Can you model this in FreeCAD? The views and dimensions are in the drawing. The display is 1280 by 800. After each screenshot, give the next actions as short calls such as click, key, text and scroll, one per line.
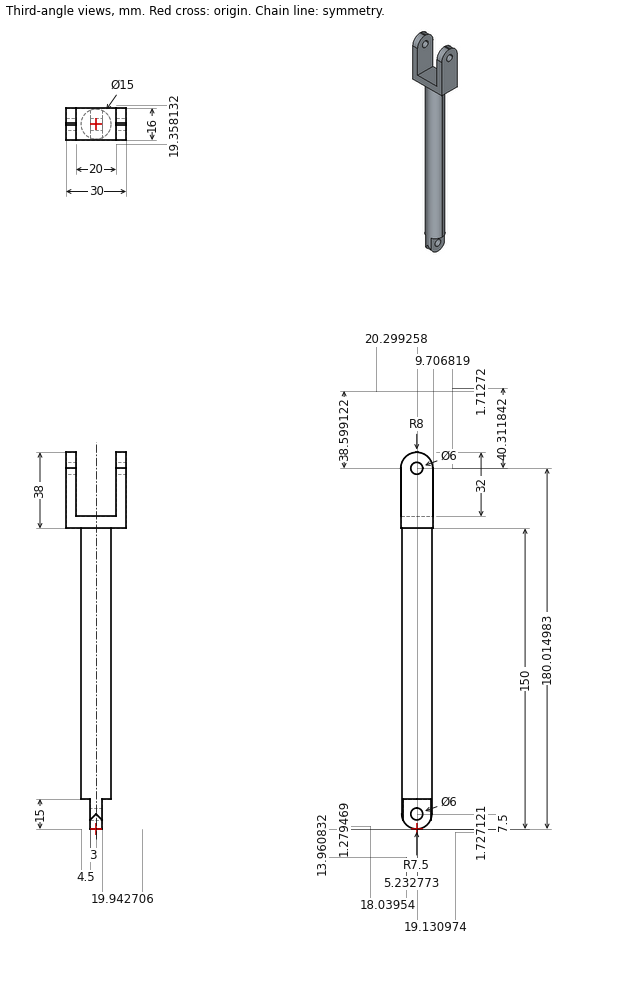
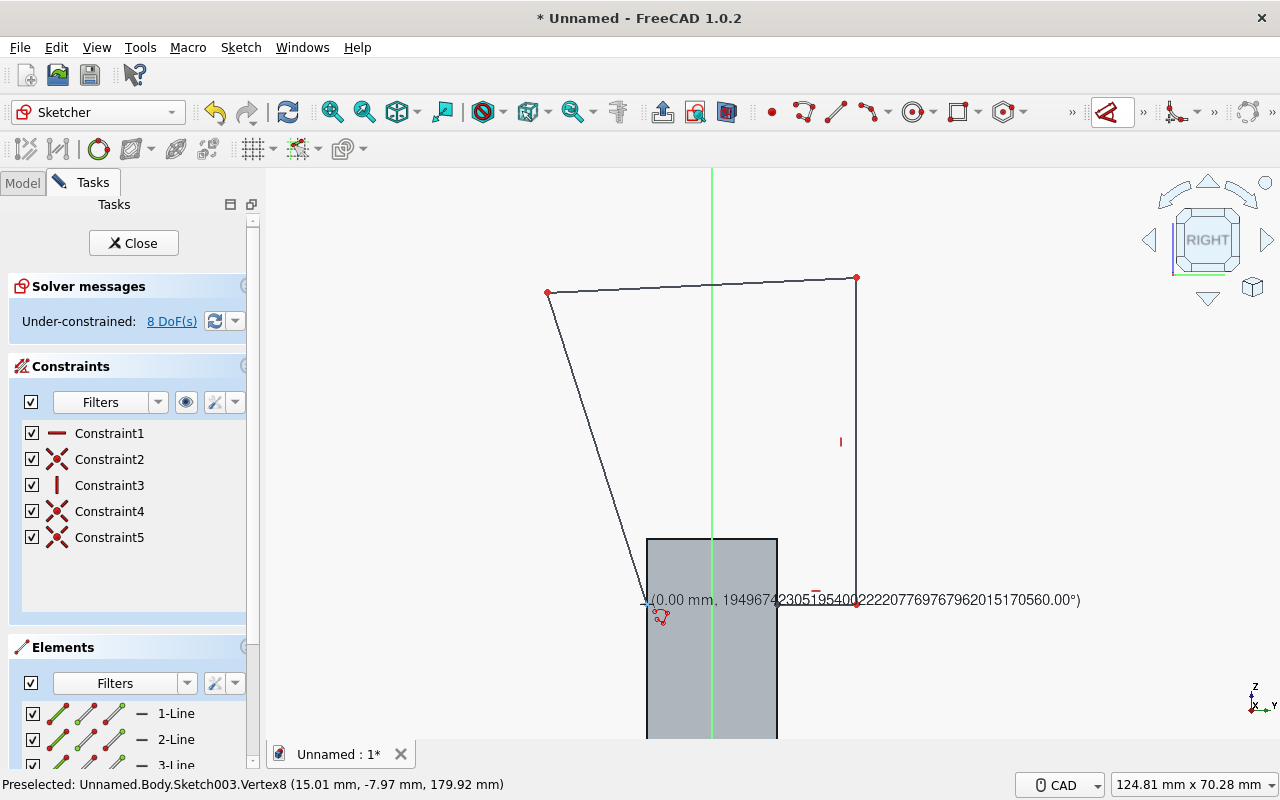
click(868, 112)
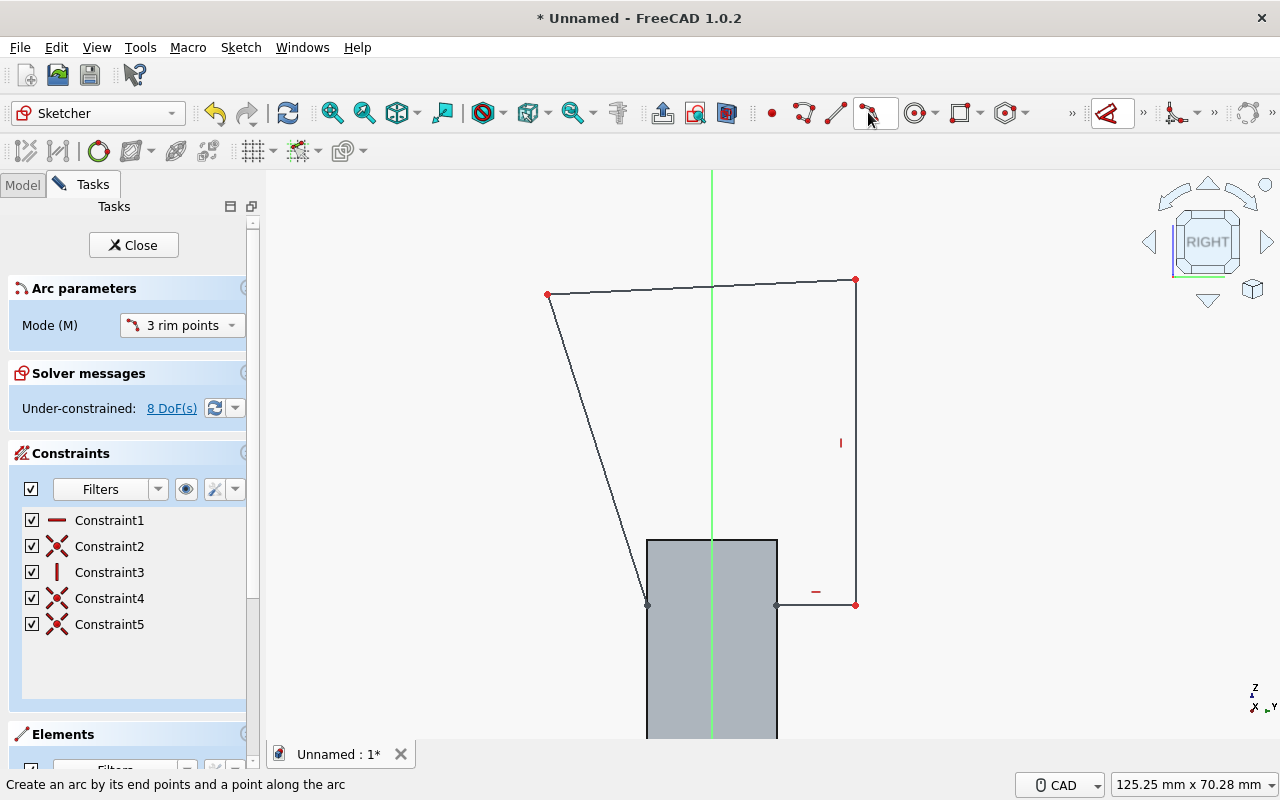
click(647, 605)
click(777, 605)
click(732, 543)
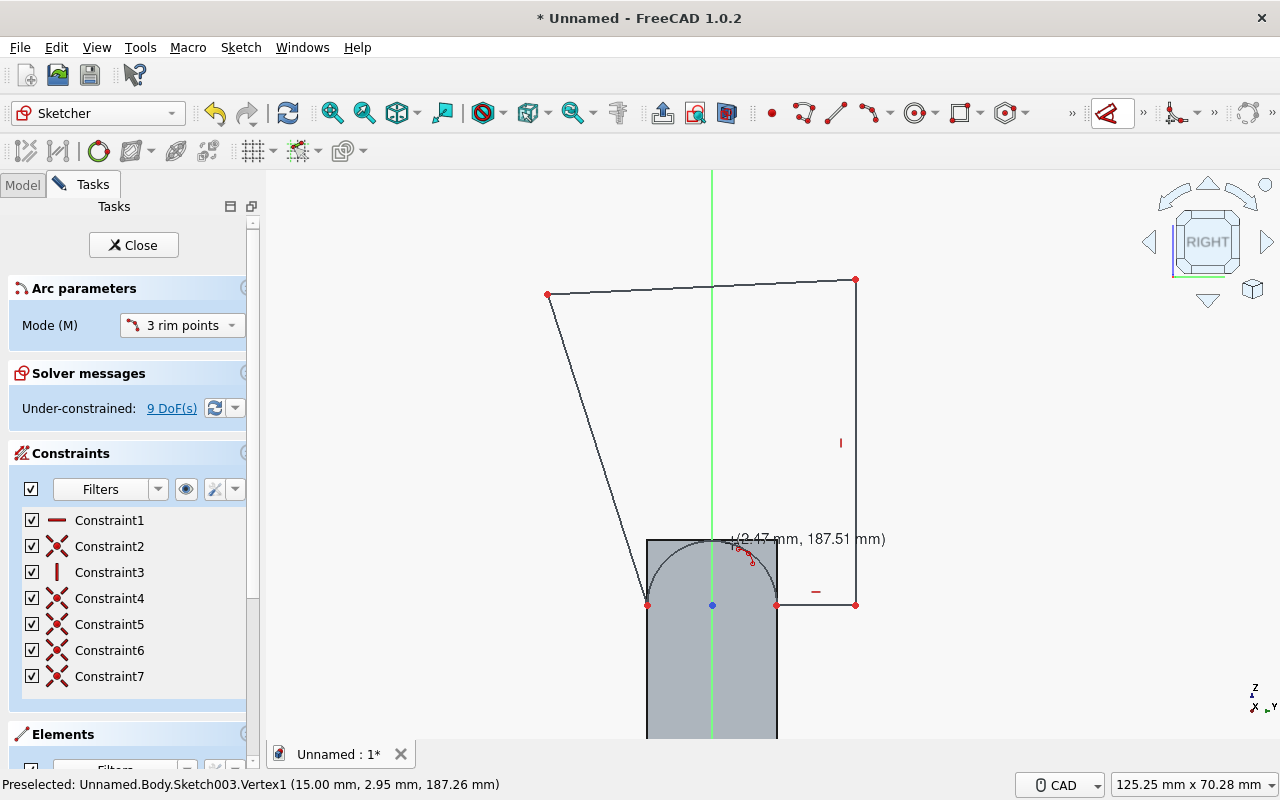
click(916, 114)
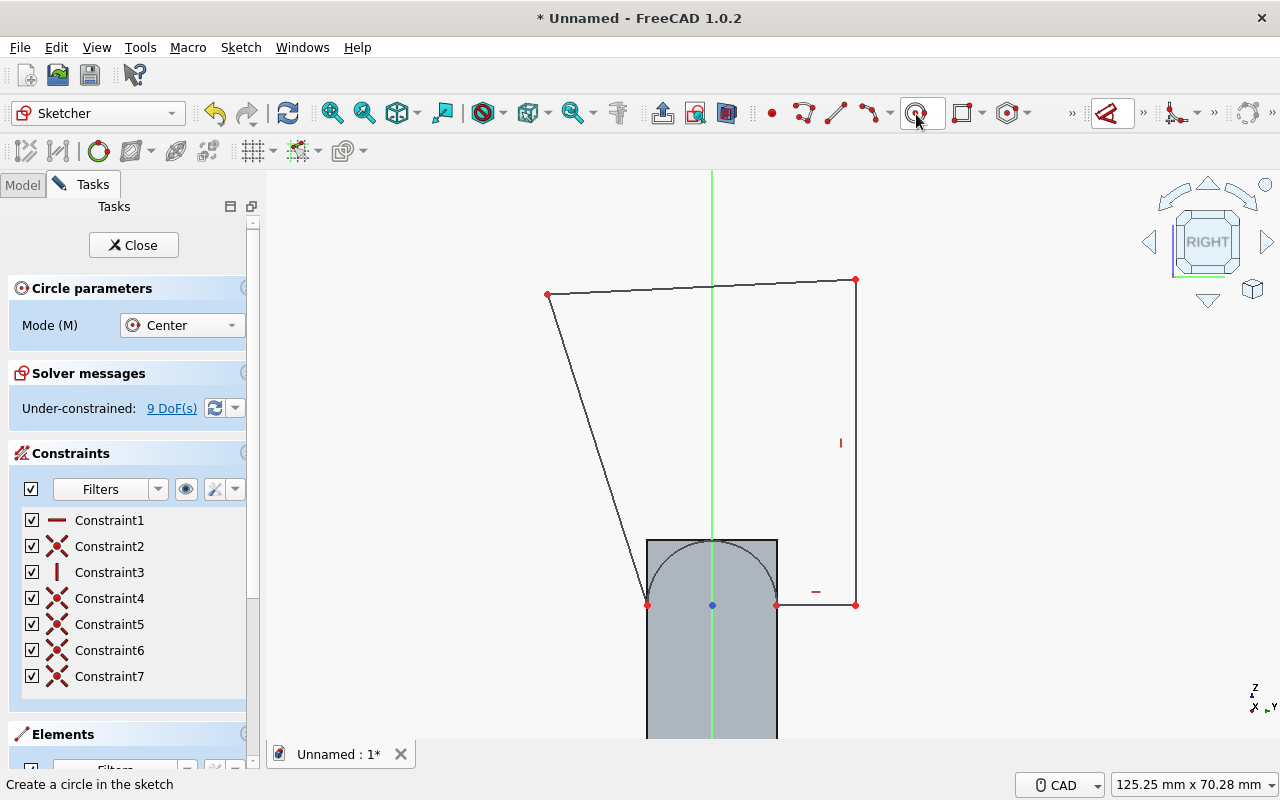
click(712, 605)
move(729, 588)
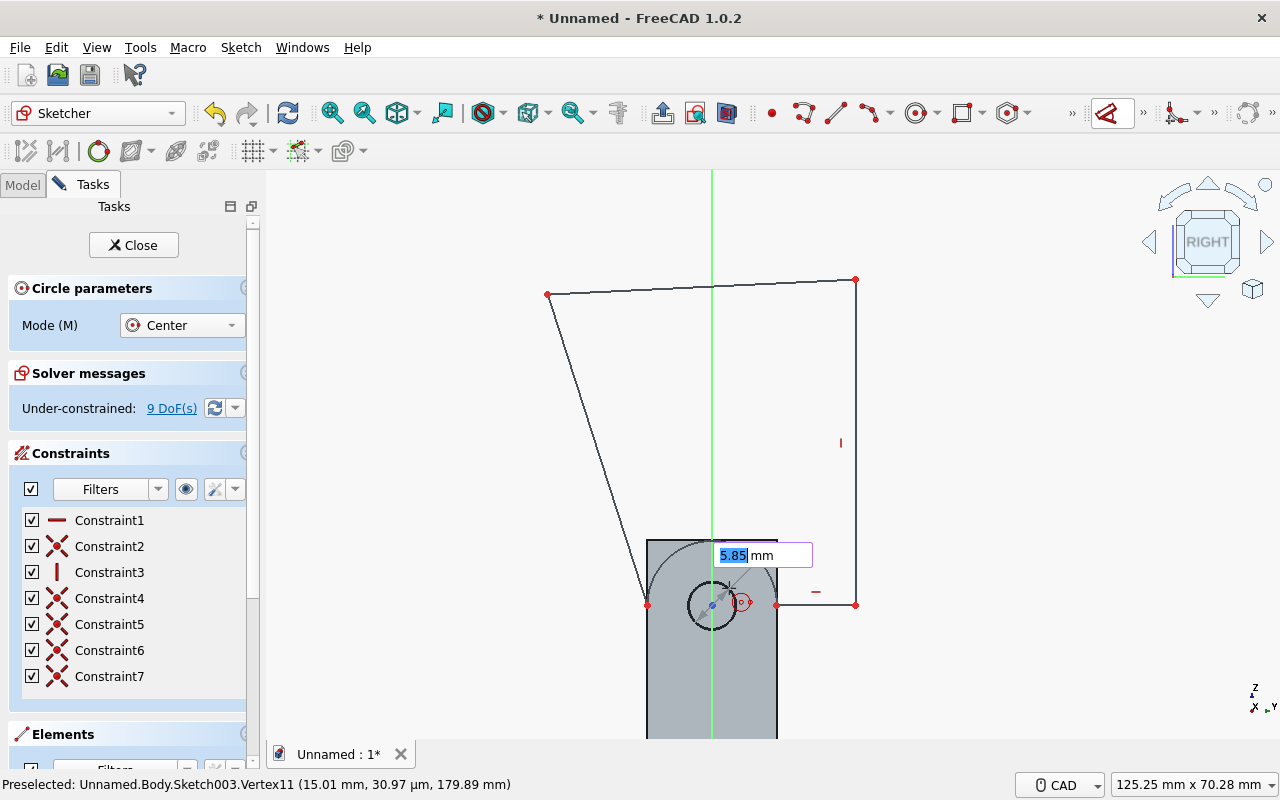
text(6)
key(Return)
key(Escape)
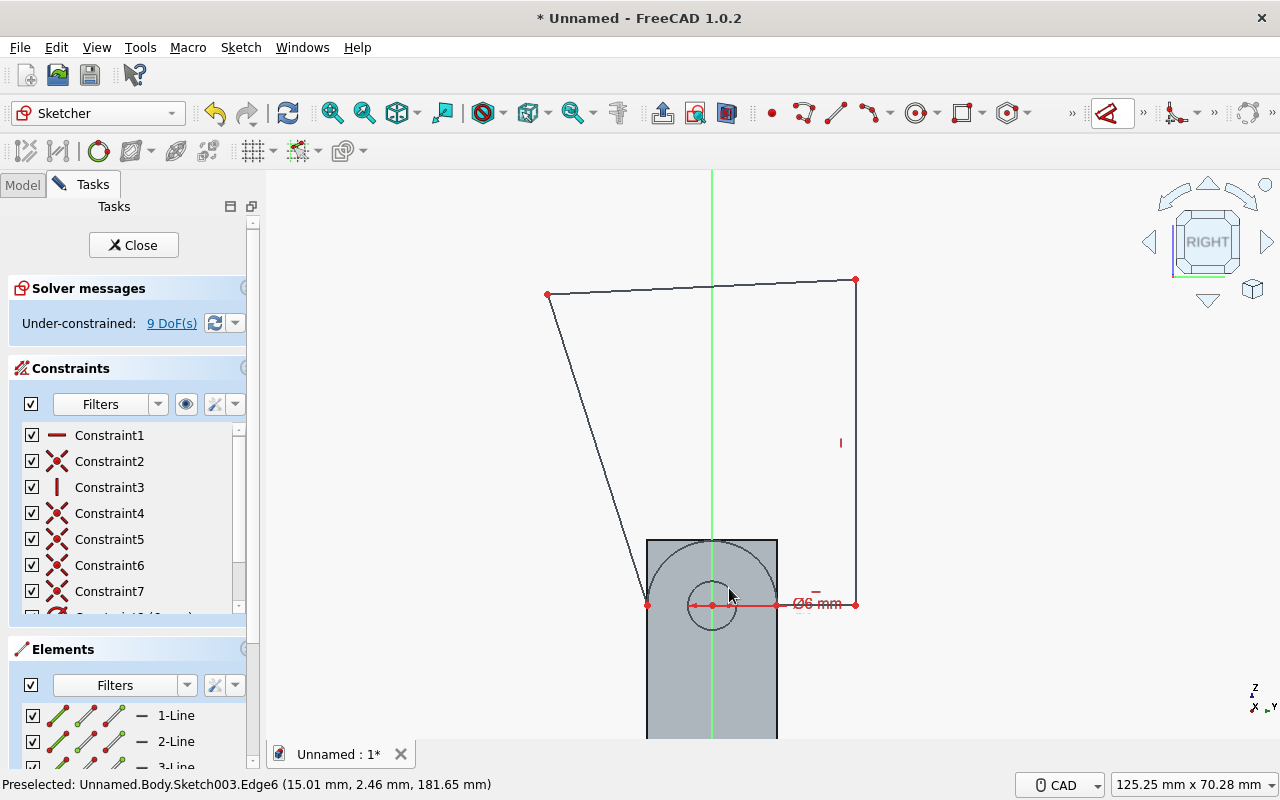
click(712, 606)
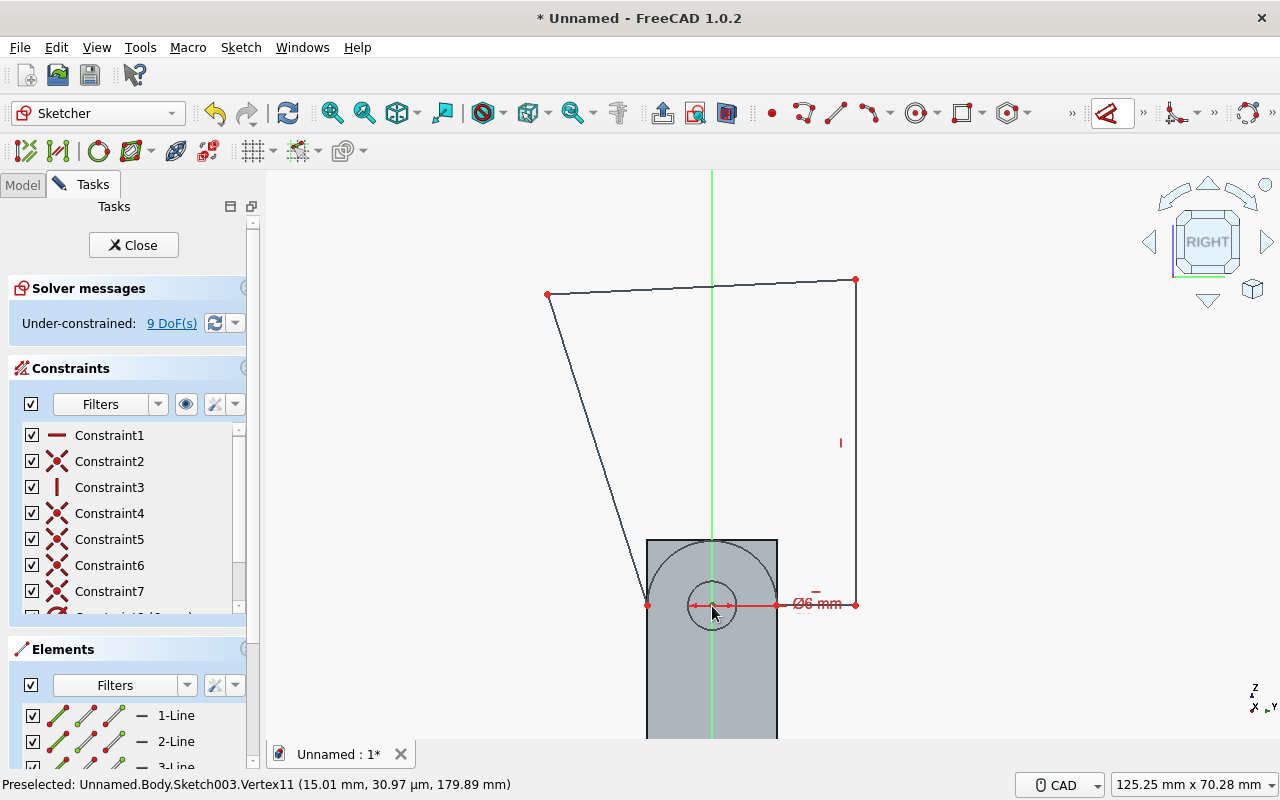
click(712, 674)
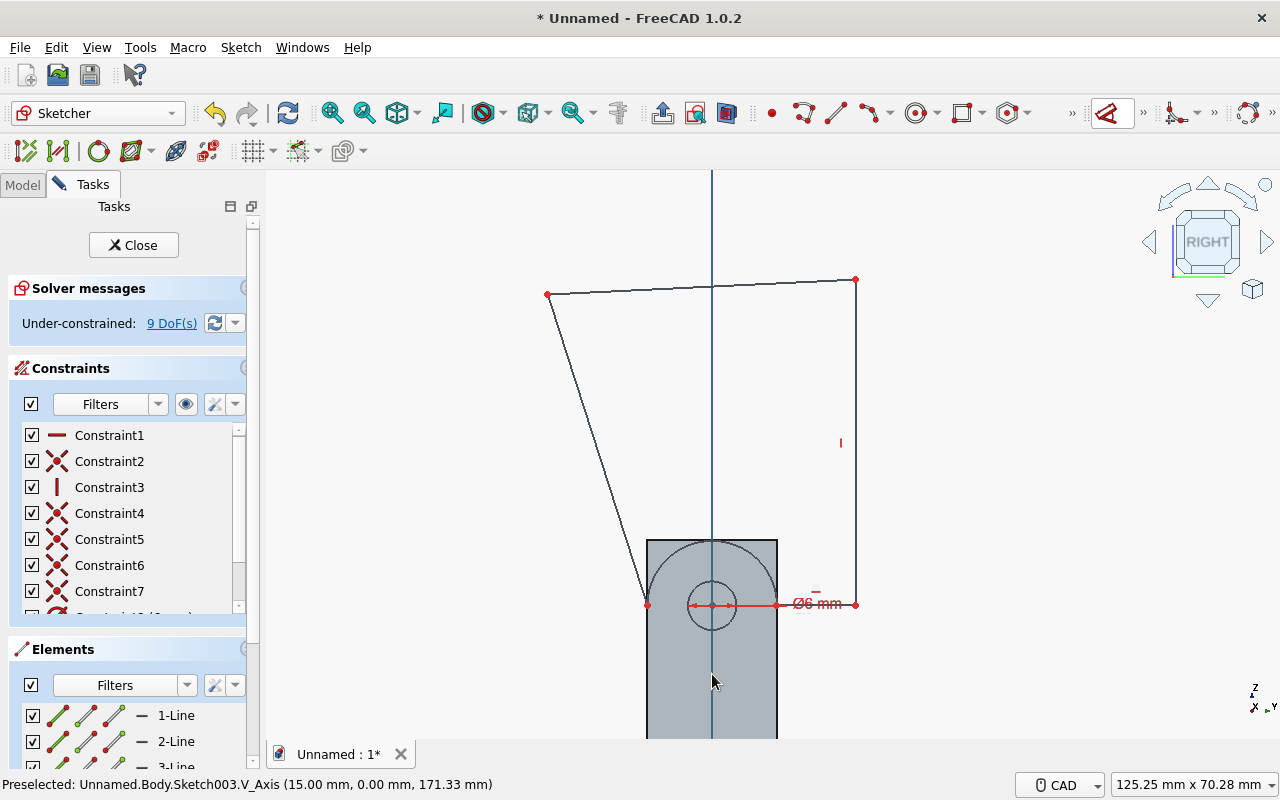
key(c)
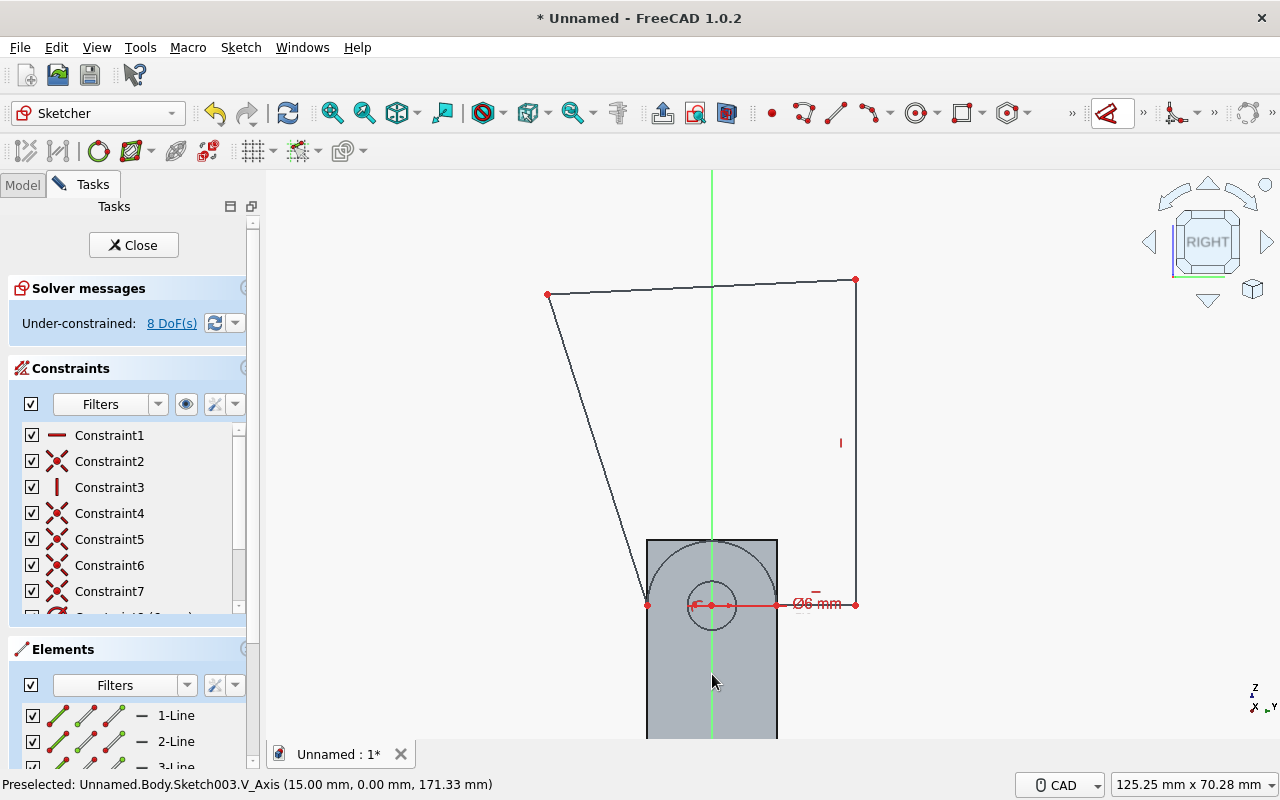
key(d)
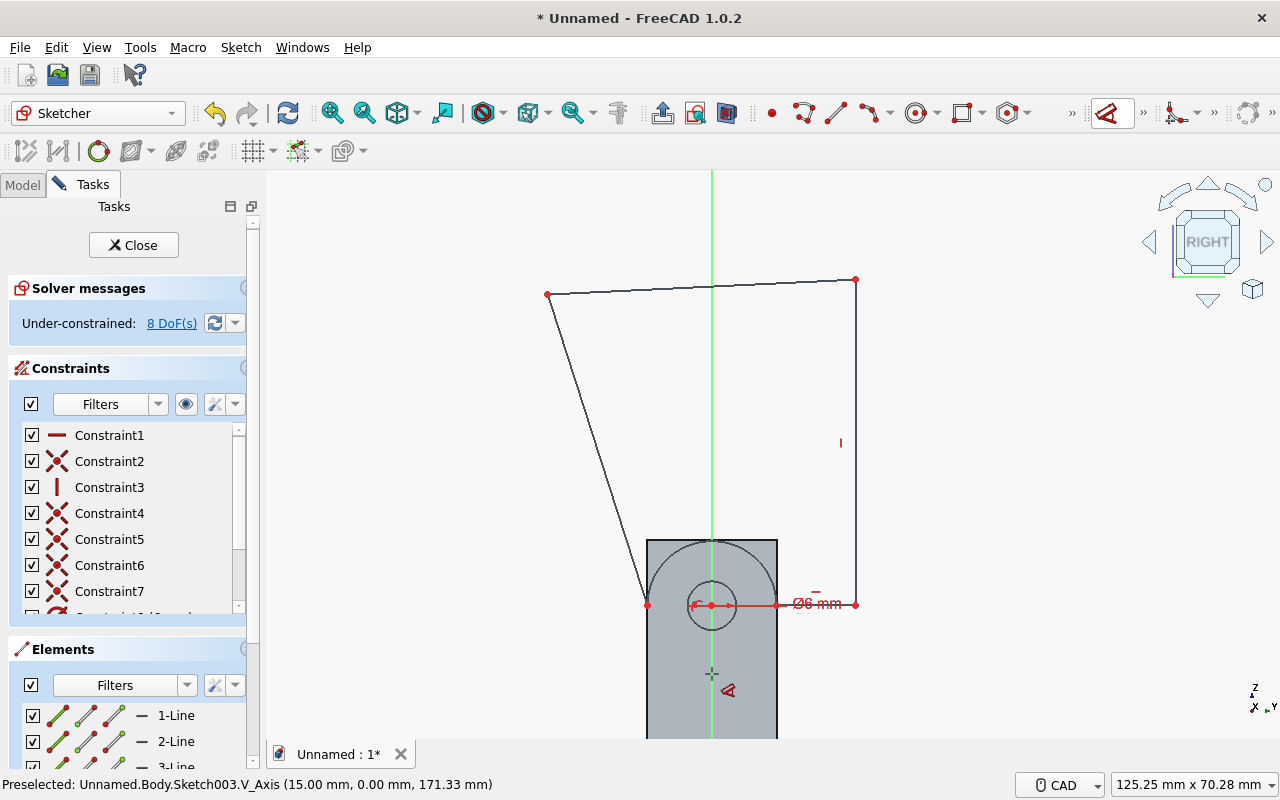
click(750, 553)
click(769, 527)